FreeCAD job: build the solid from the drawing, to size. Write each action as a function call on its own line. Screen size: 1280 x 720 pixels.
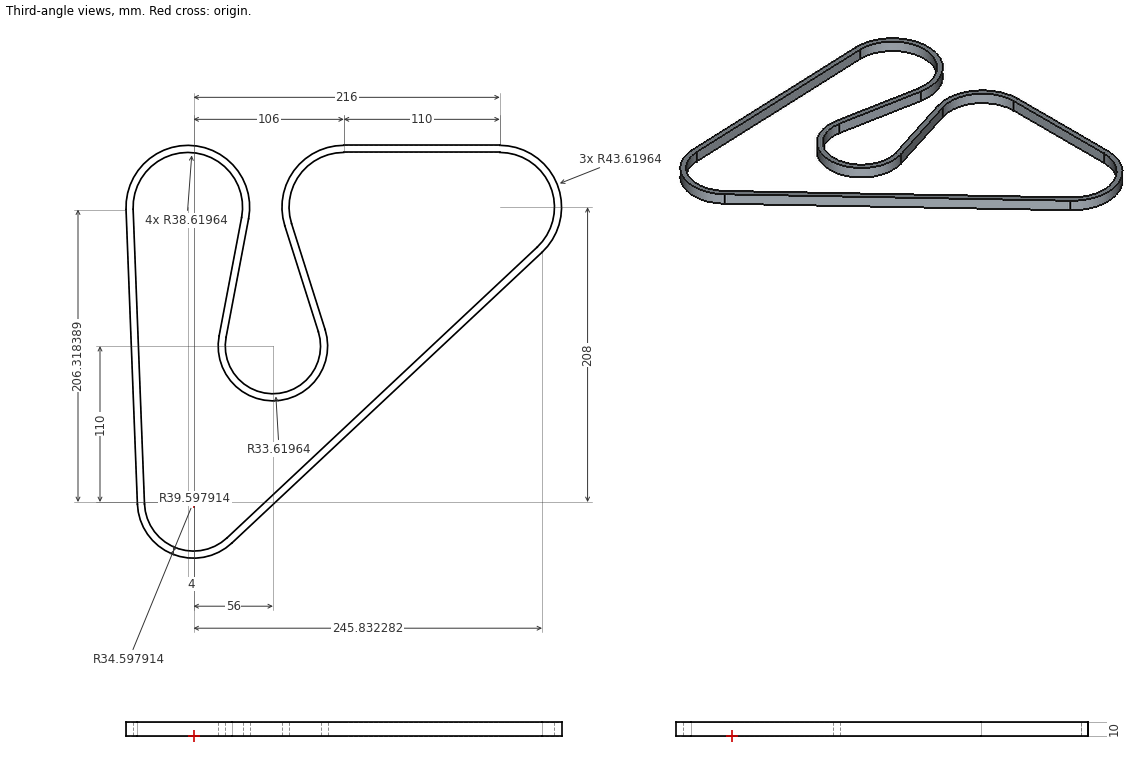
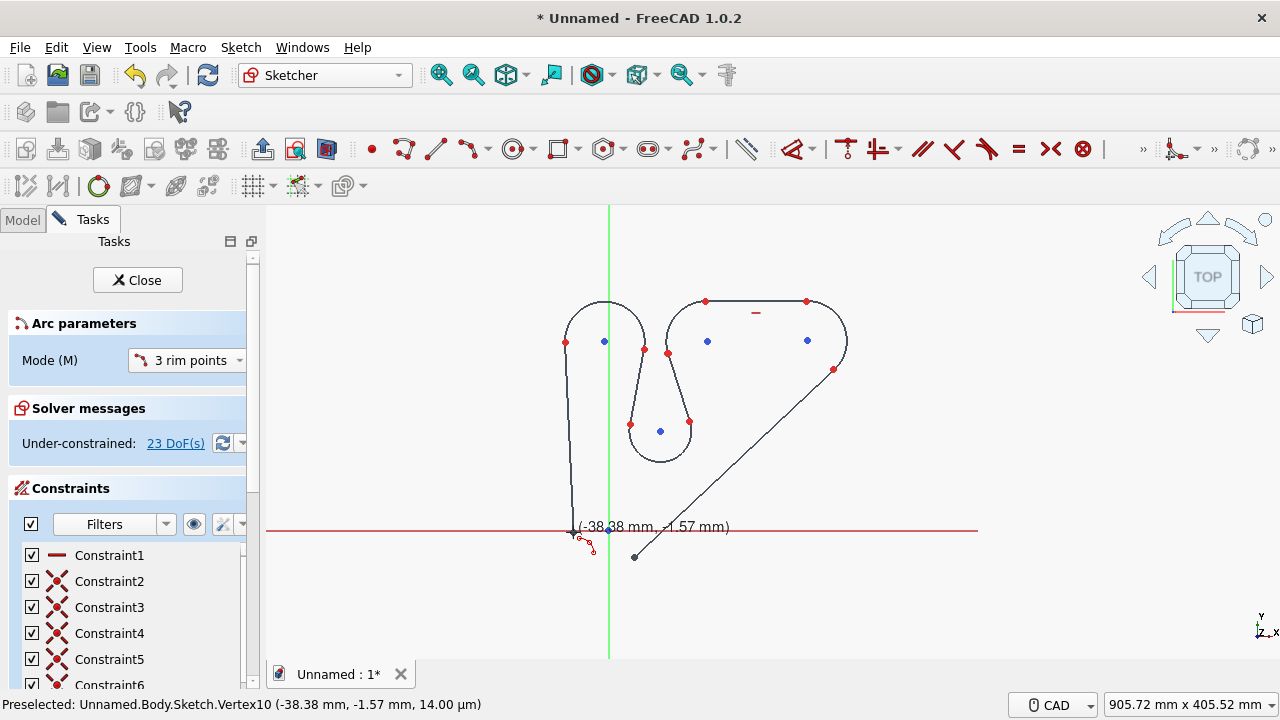
click(634, 558)
click(588, 560)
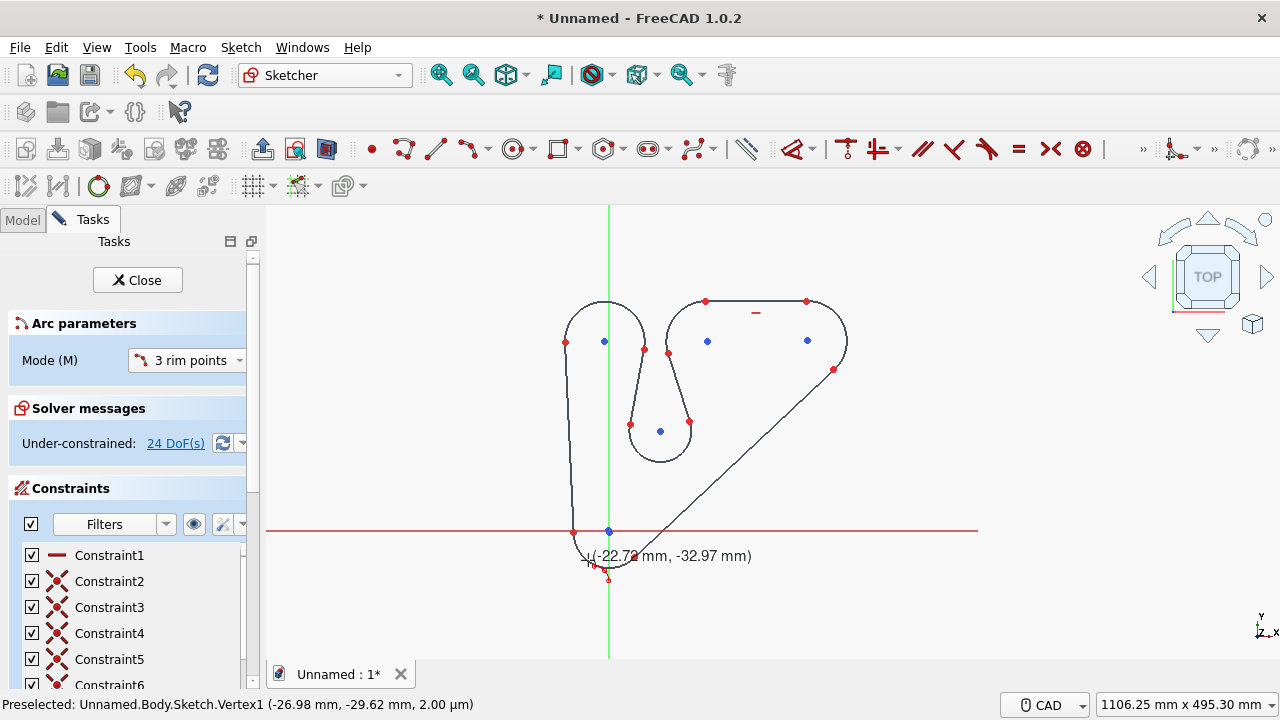
key(g)
key(l)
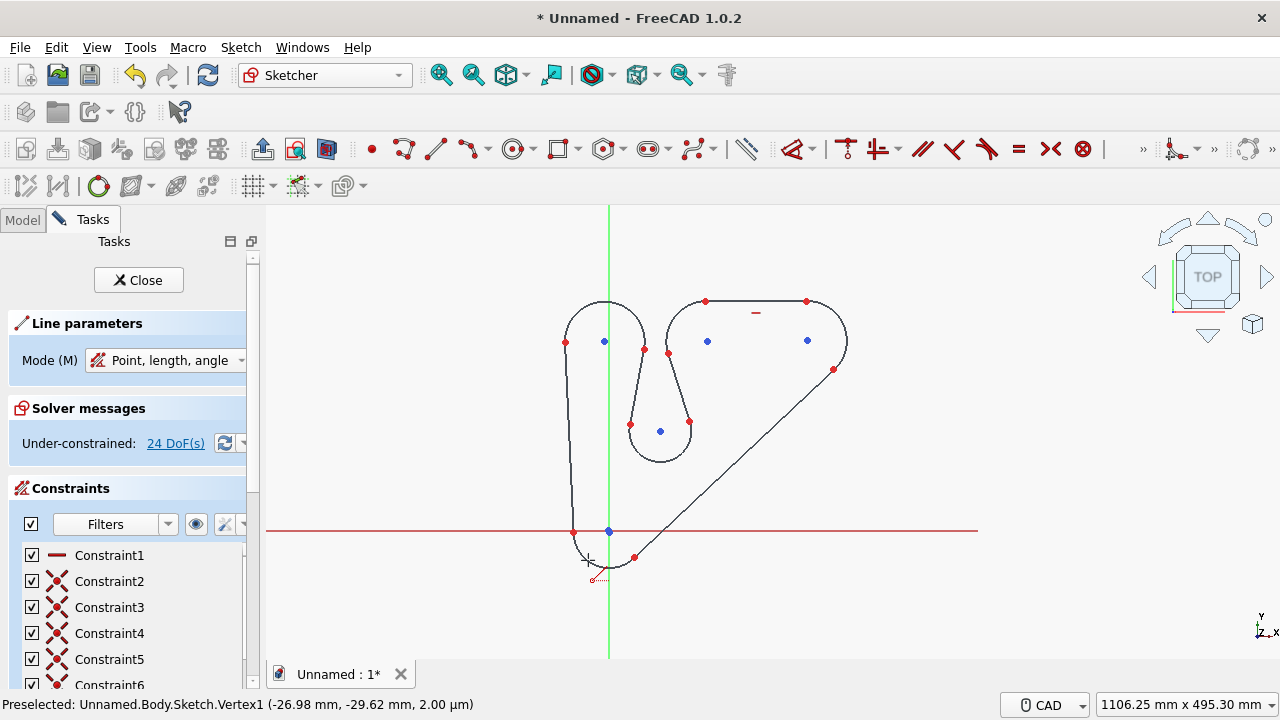
scroll(831, 366, up, 7)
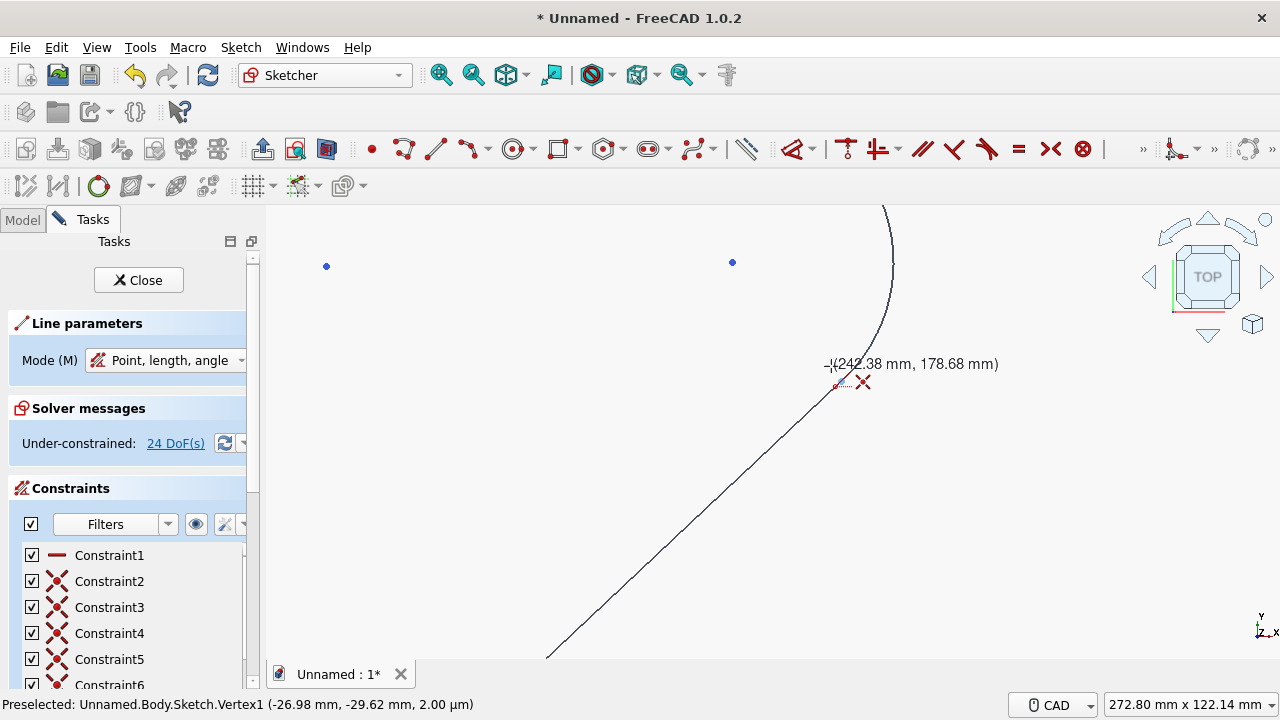
click(829, 365)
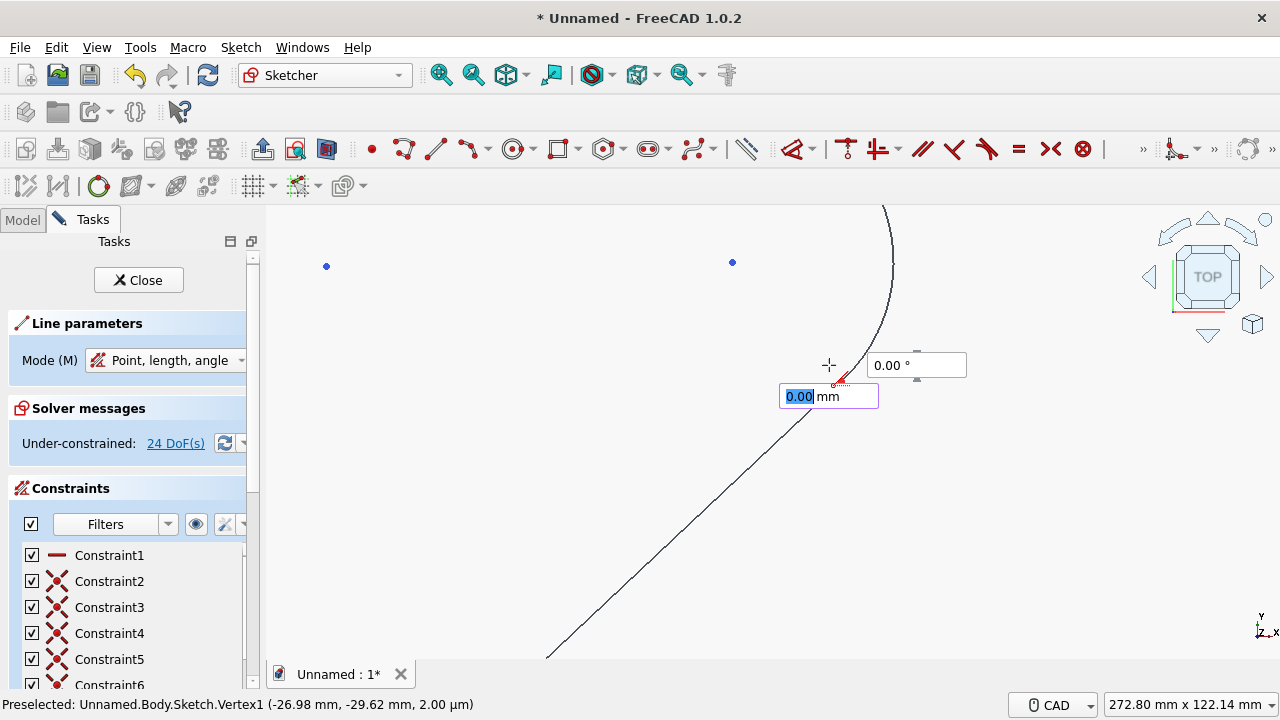
scroll(831, 366, down, 7)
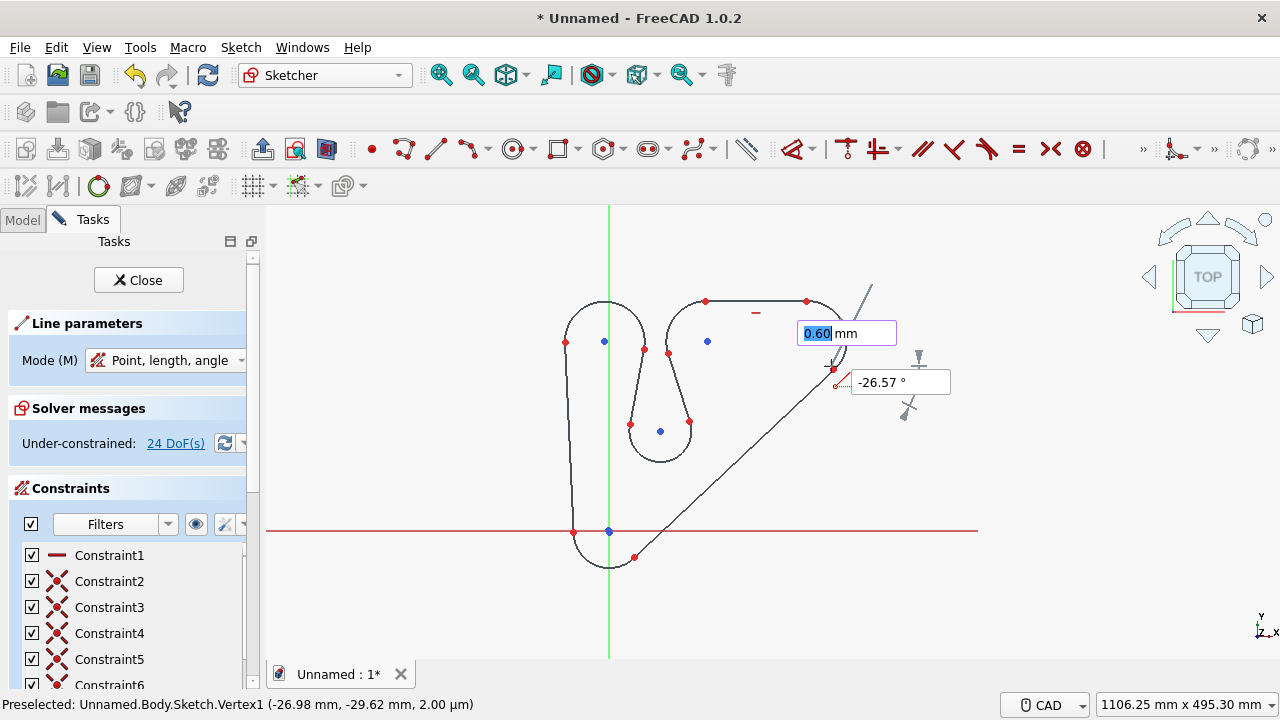
scroll(631, 554, up, 7)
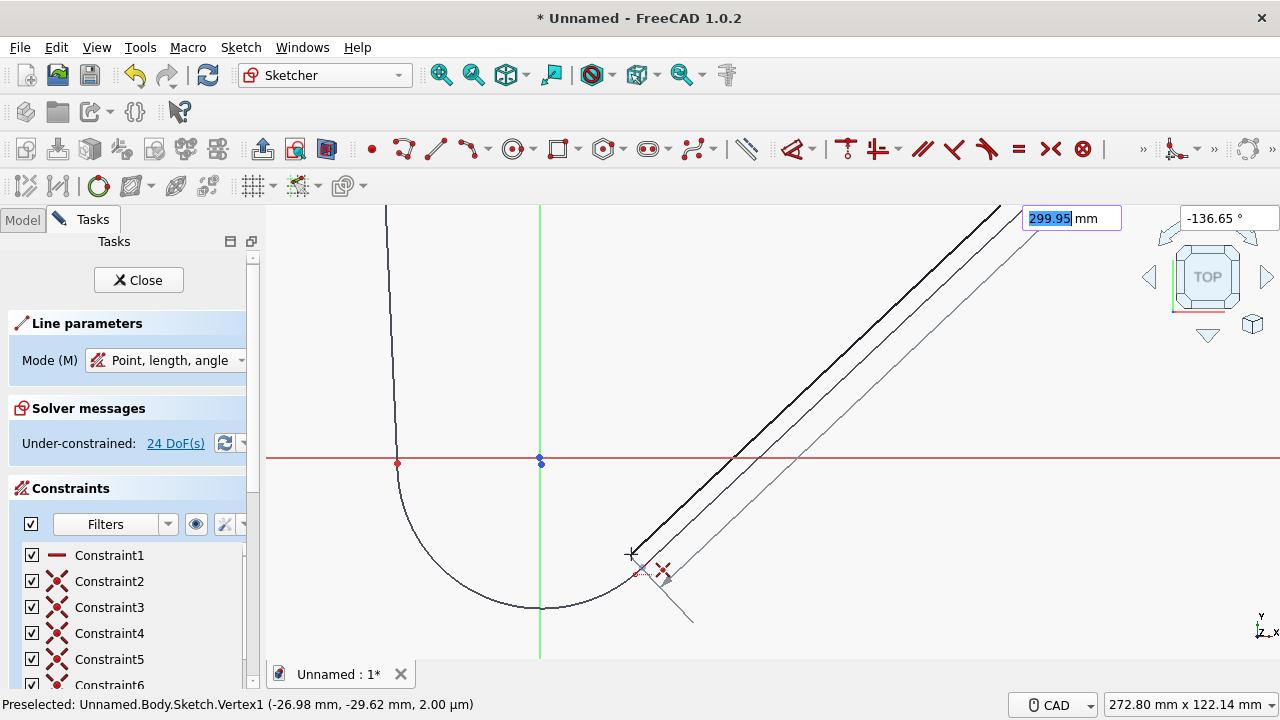
click(628, 551)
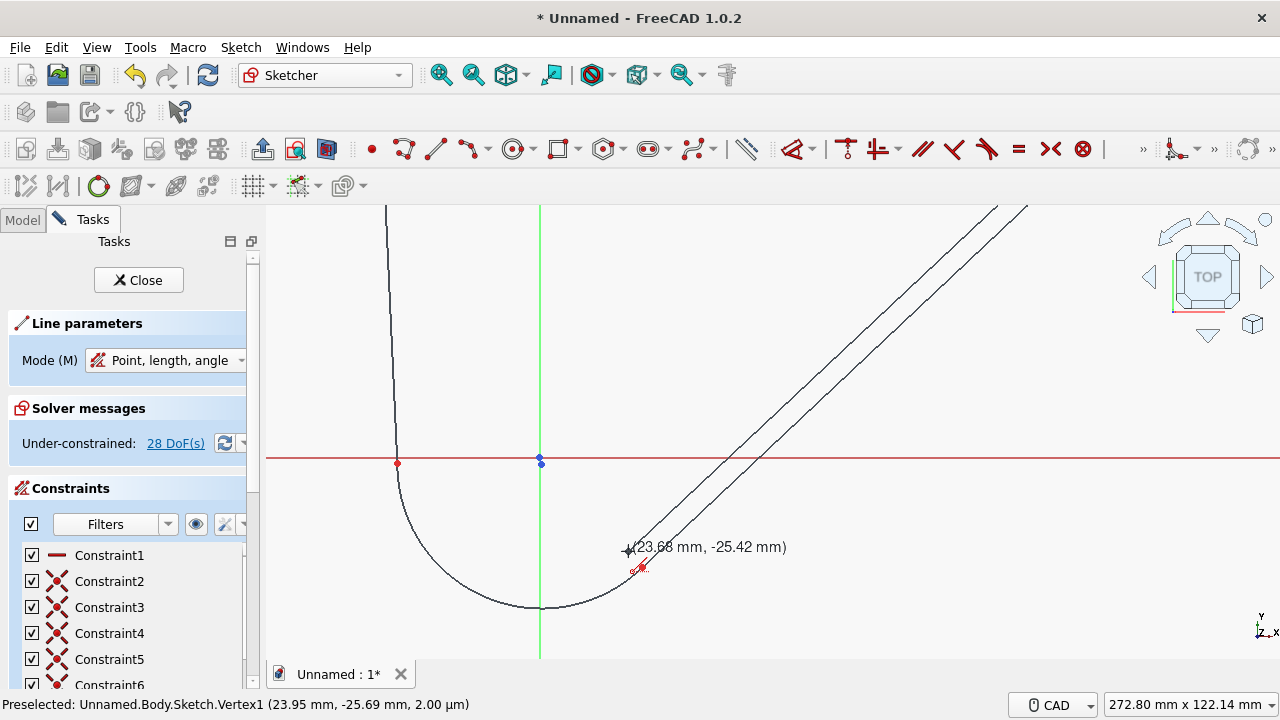
scroll(411, 462, up, 6)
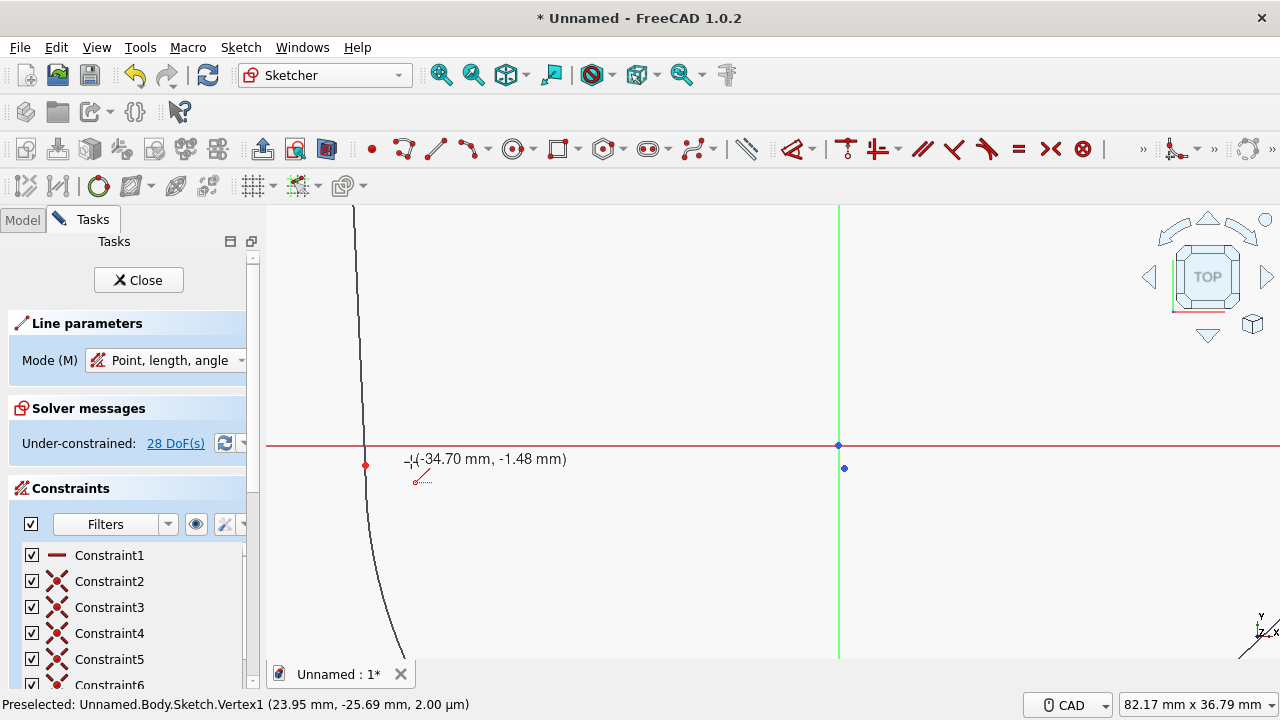
click(412, 462)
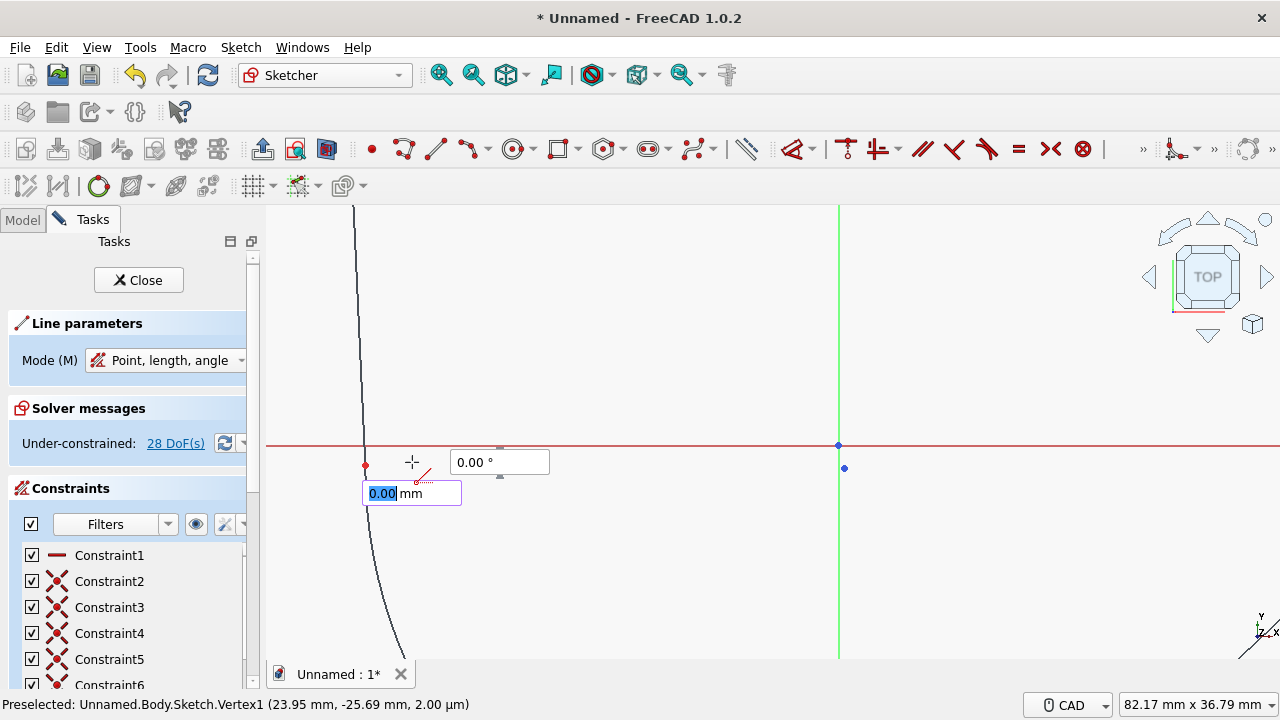
scroll(590, 537, down, 13)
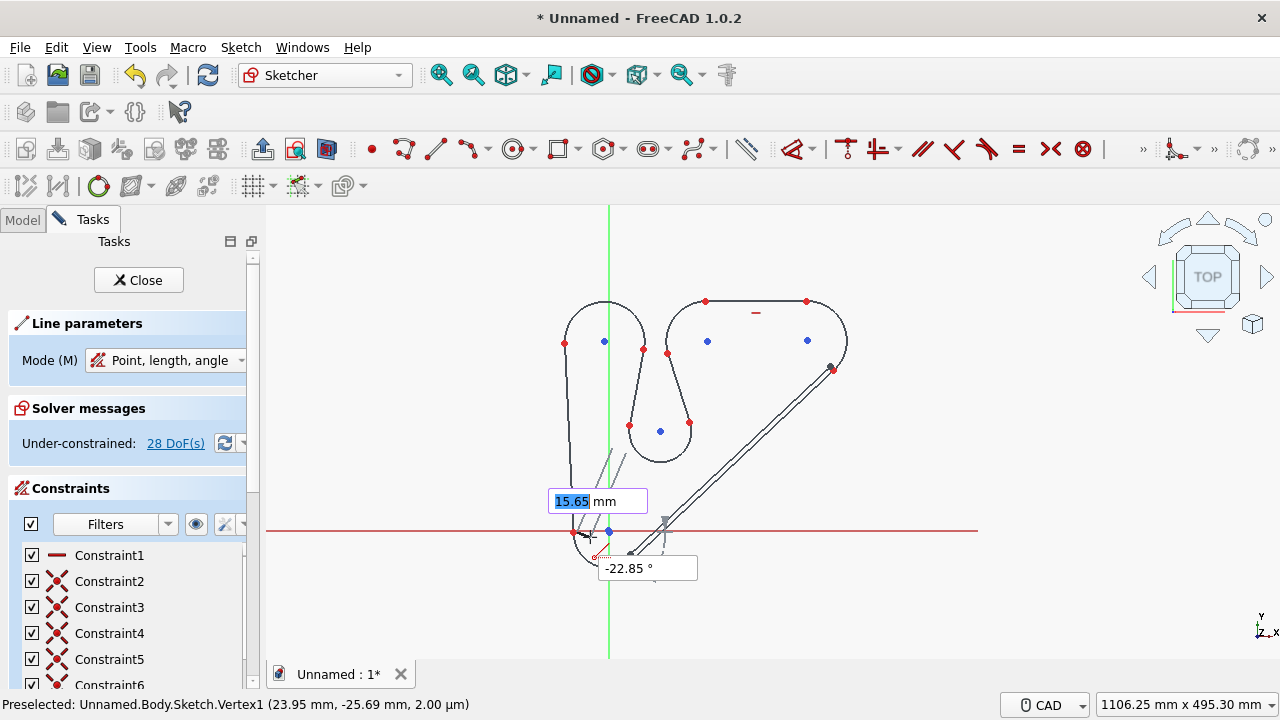
scroll(570, 342, up, 7)